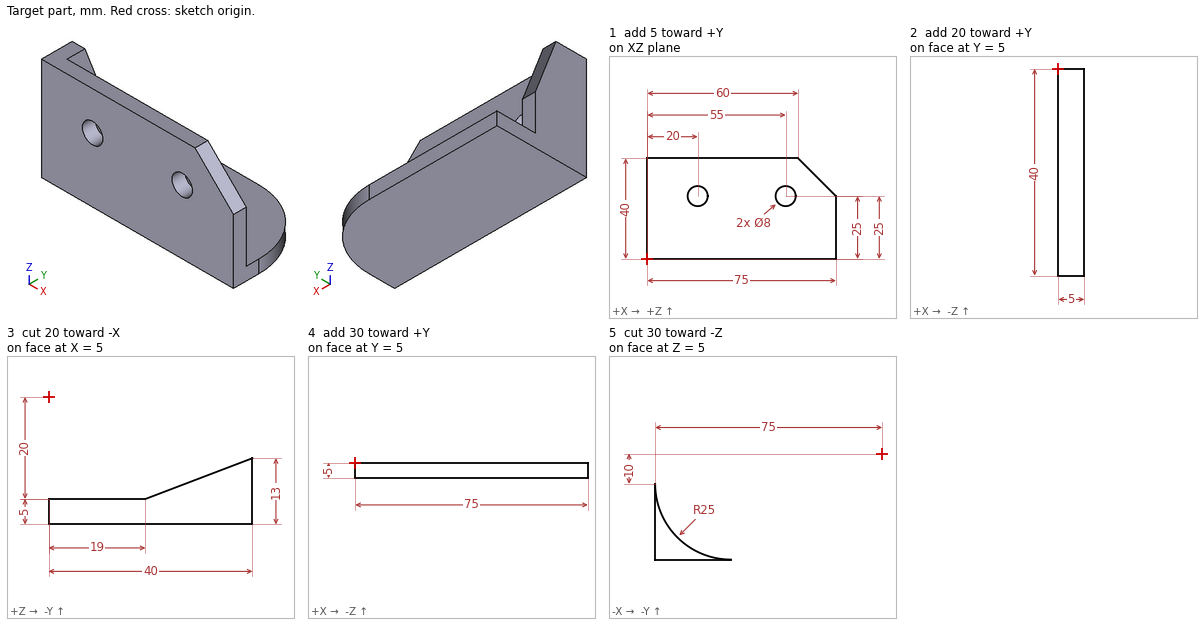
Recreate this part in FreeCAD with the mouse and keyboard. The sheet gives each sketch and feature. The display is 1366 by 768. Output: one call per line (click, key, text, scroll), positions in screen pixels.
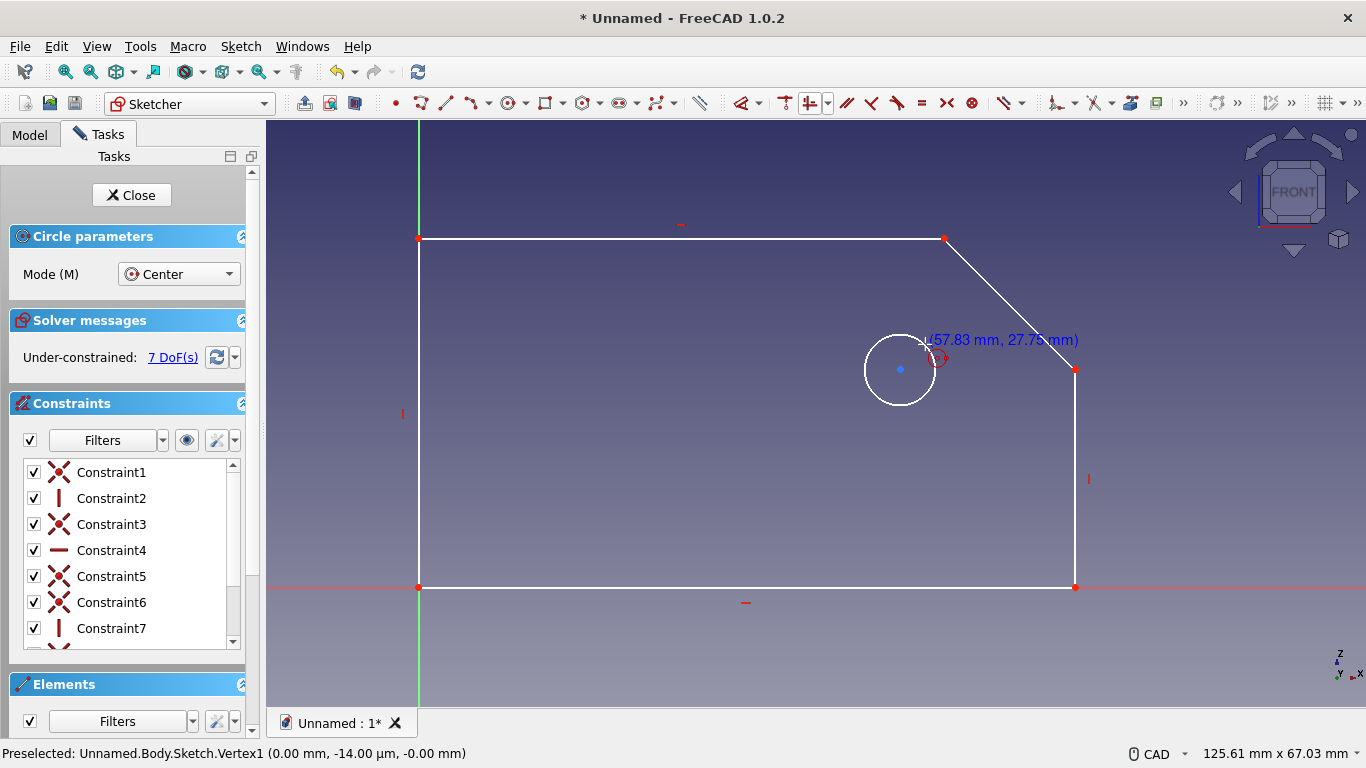
click(594, 369)
click(618, 344)
key(Escape)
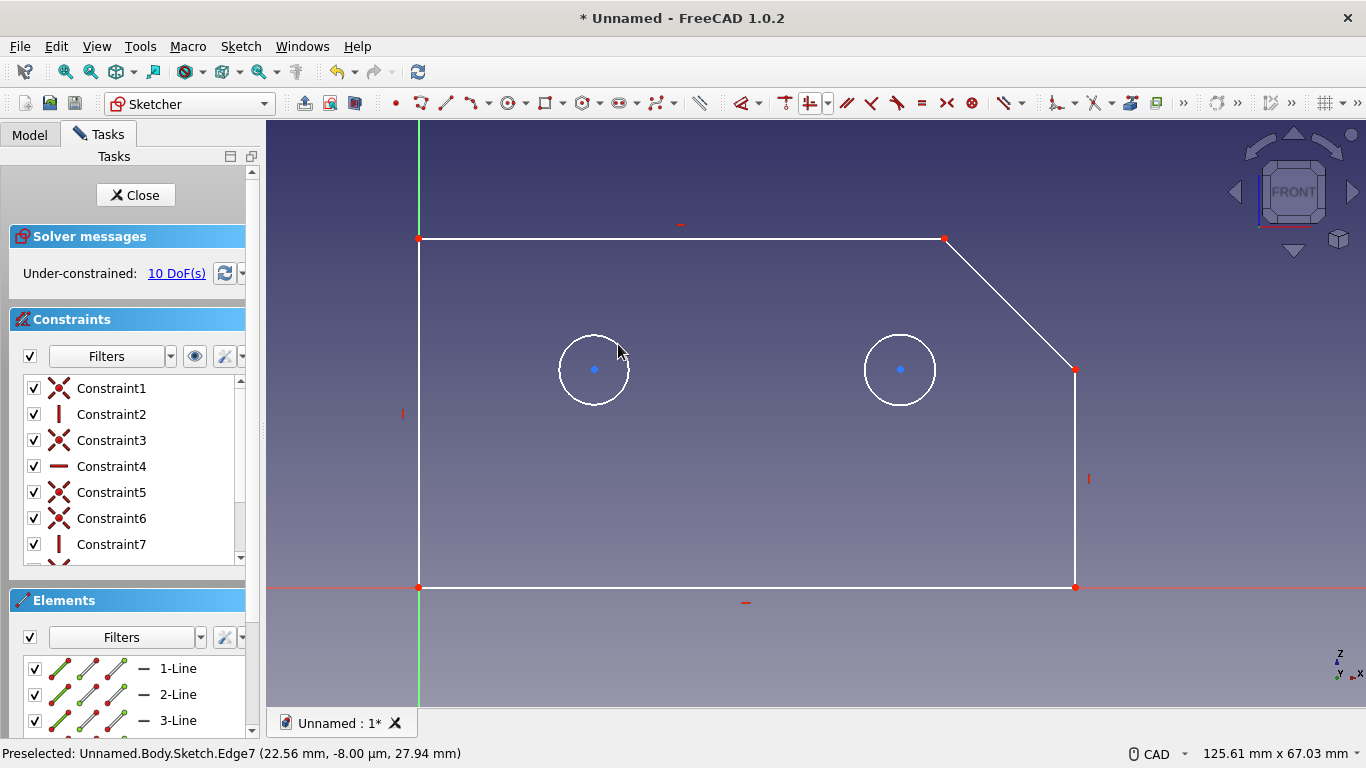
click(925, 345)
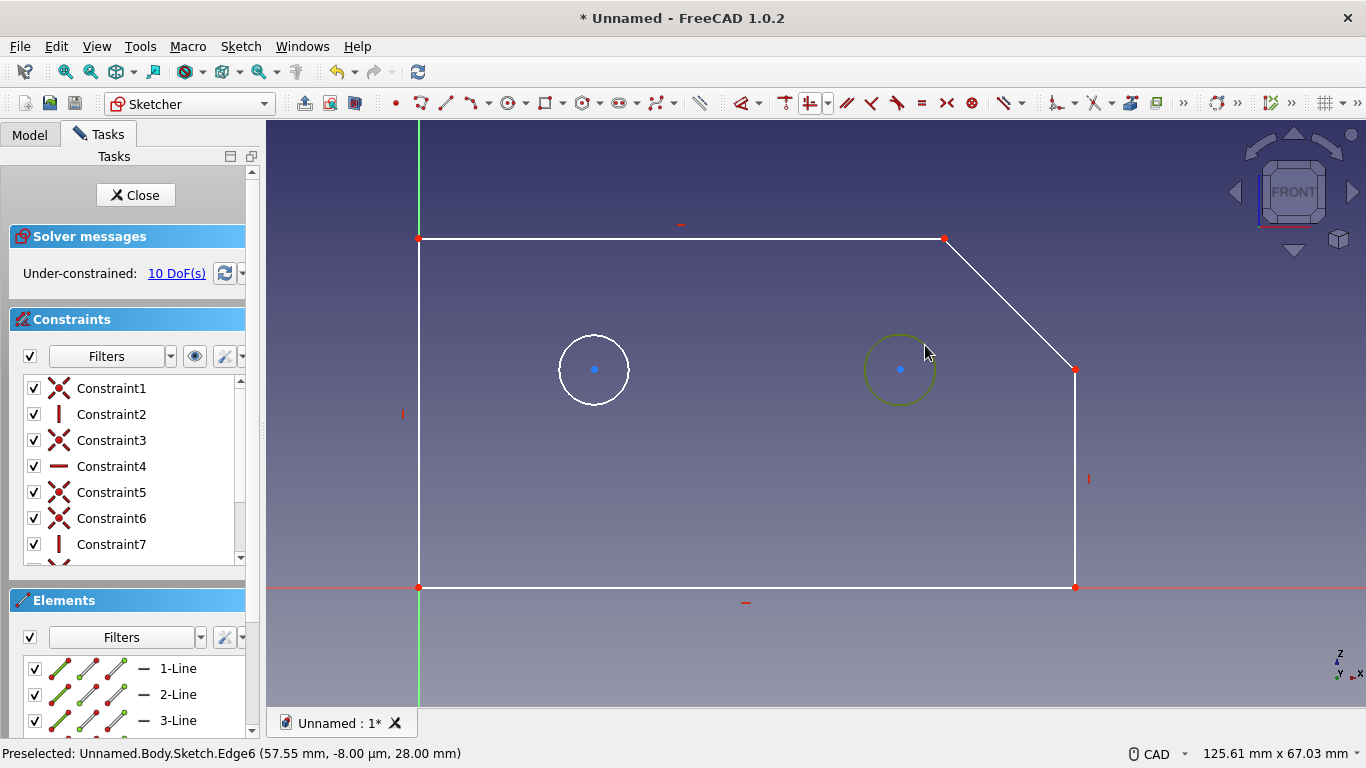
click(618, 345)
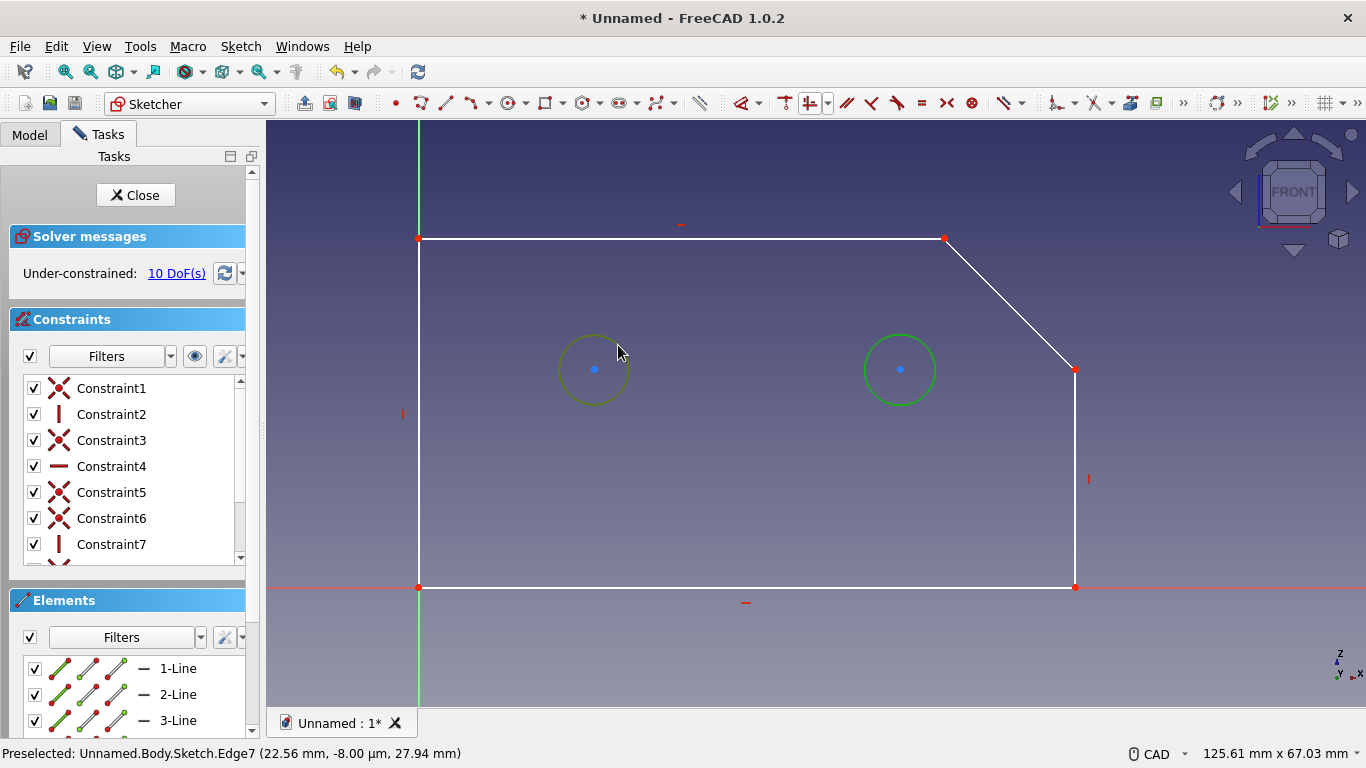
click(922, 104)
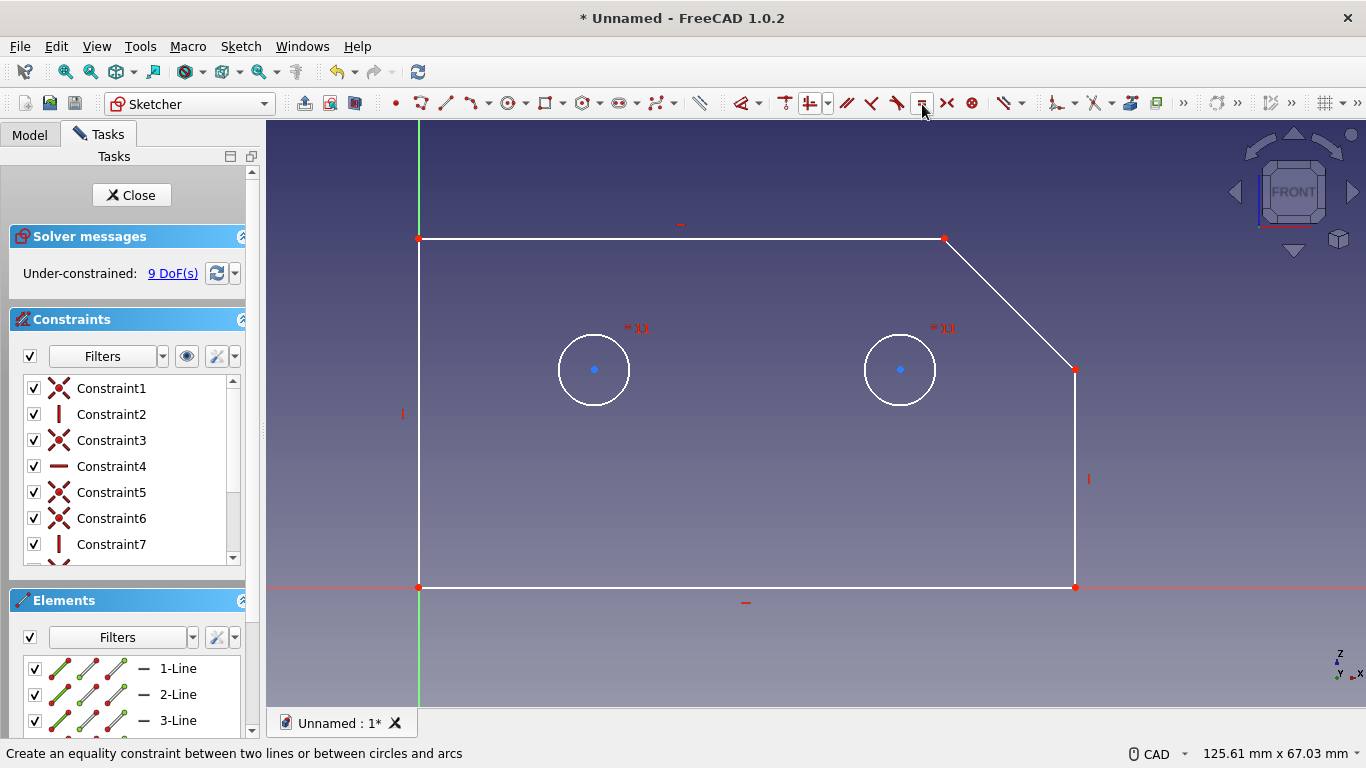
click(900, 370)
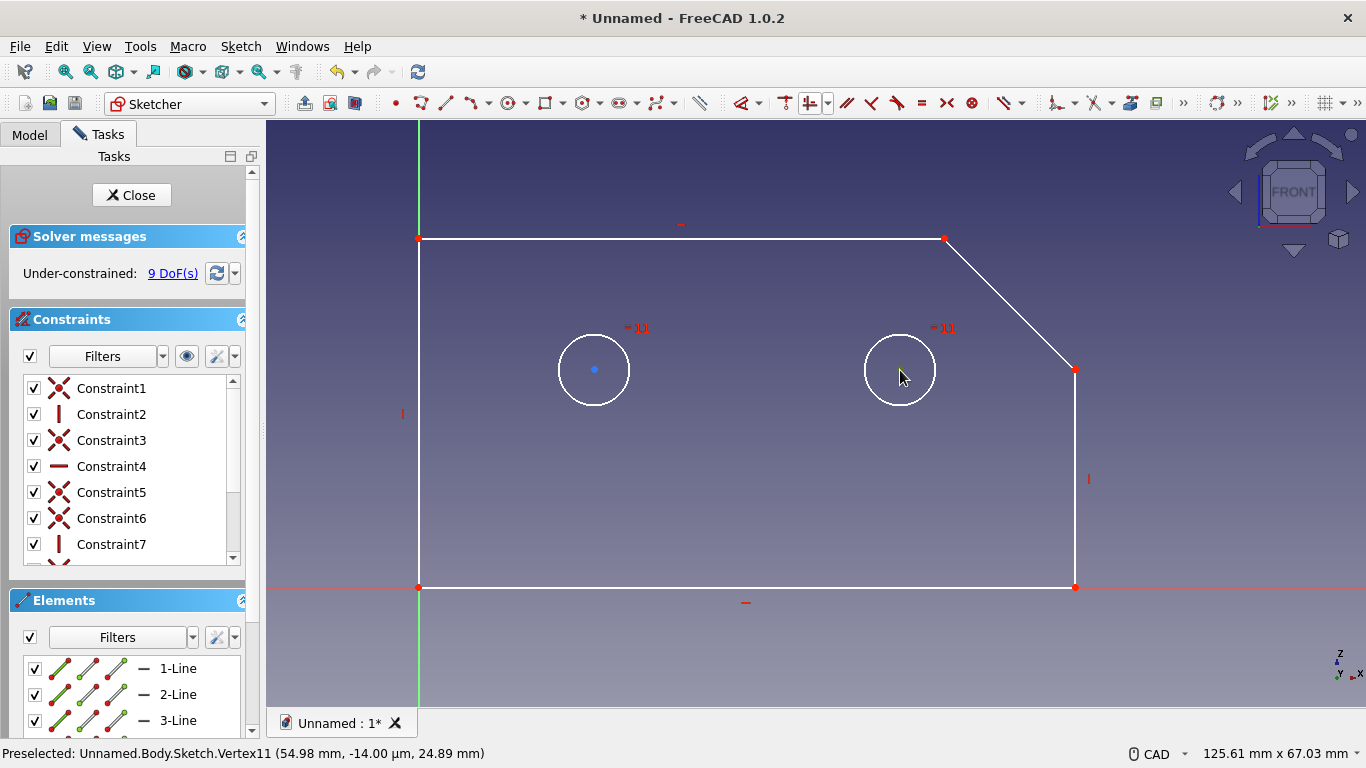
click(594, 370)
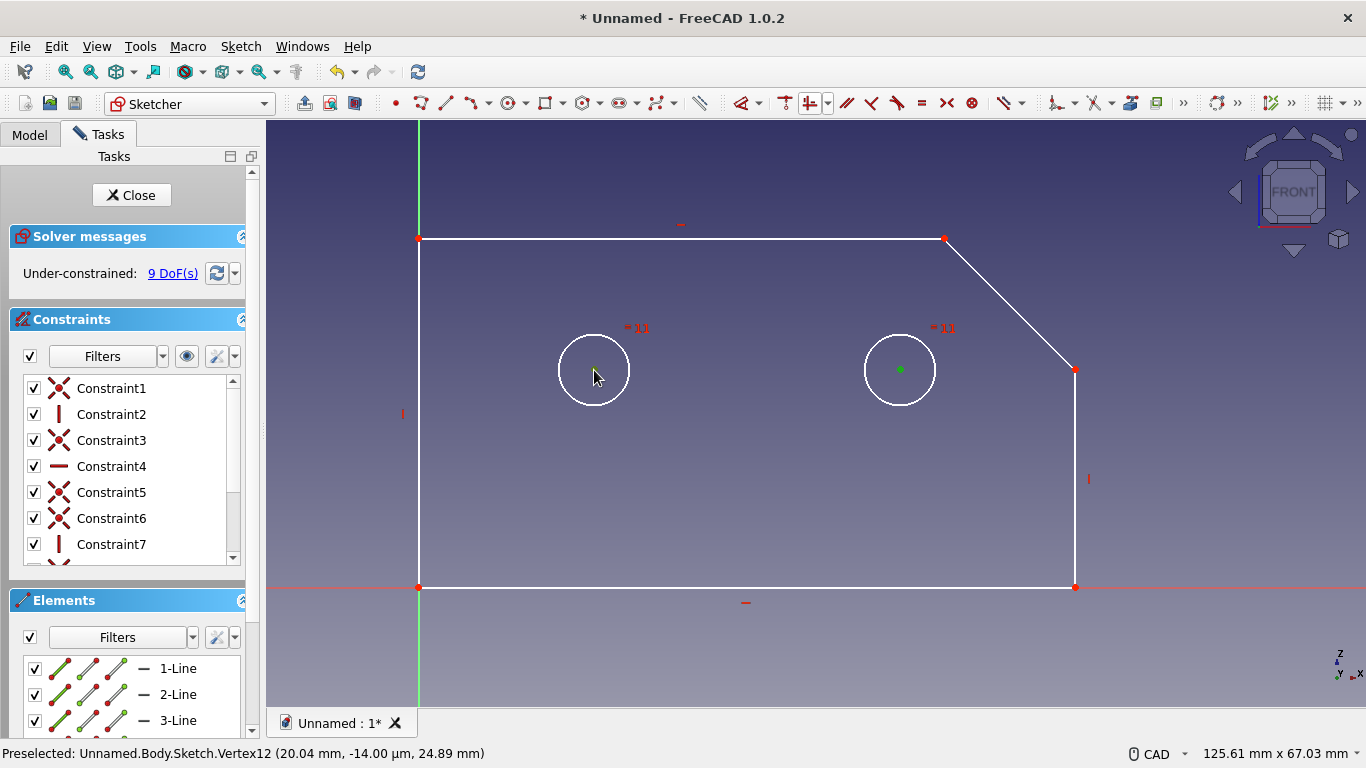
key(h)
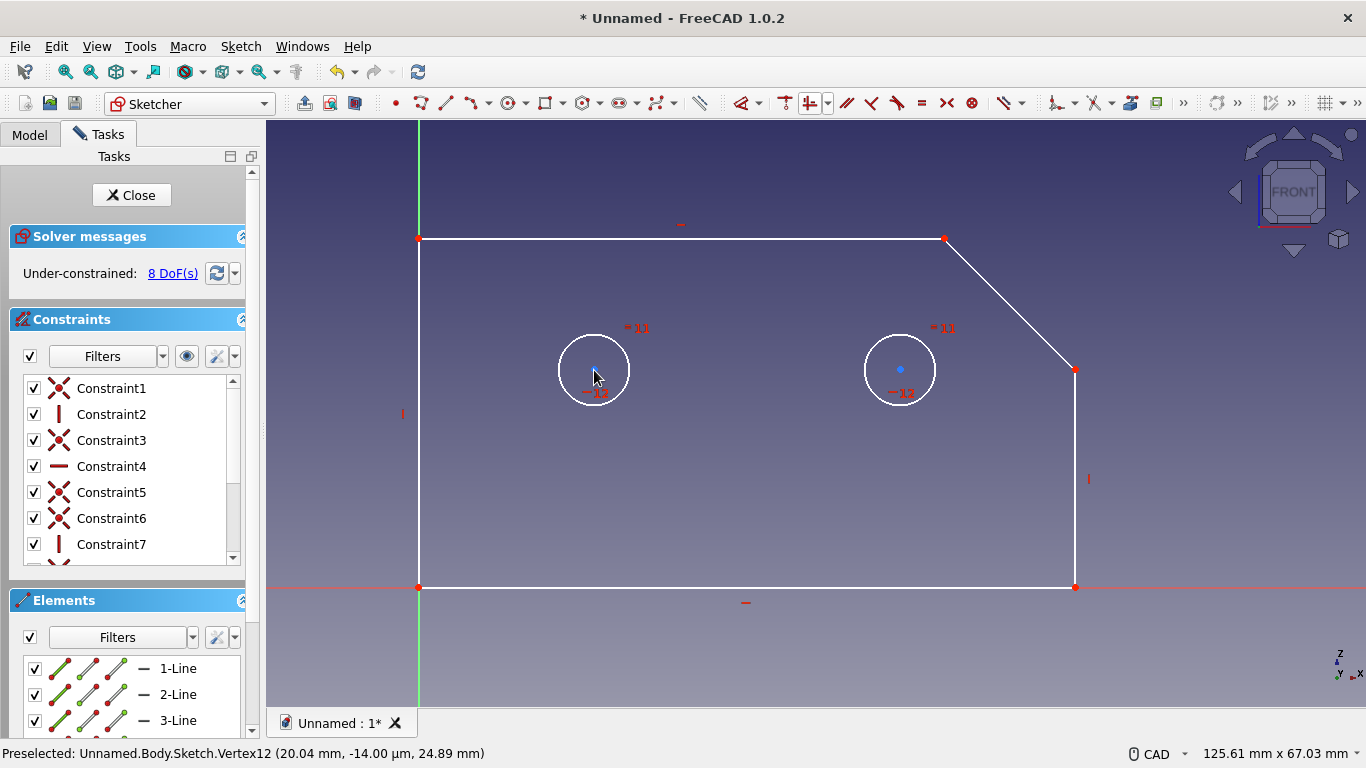
click(740, 104)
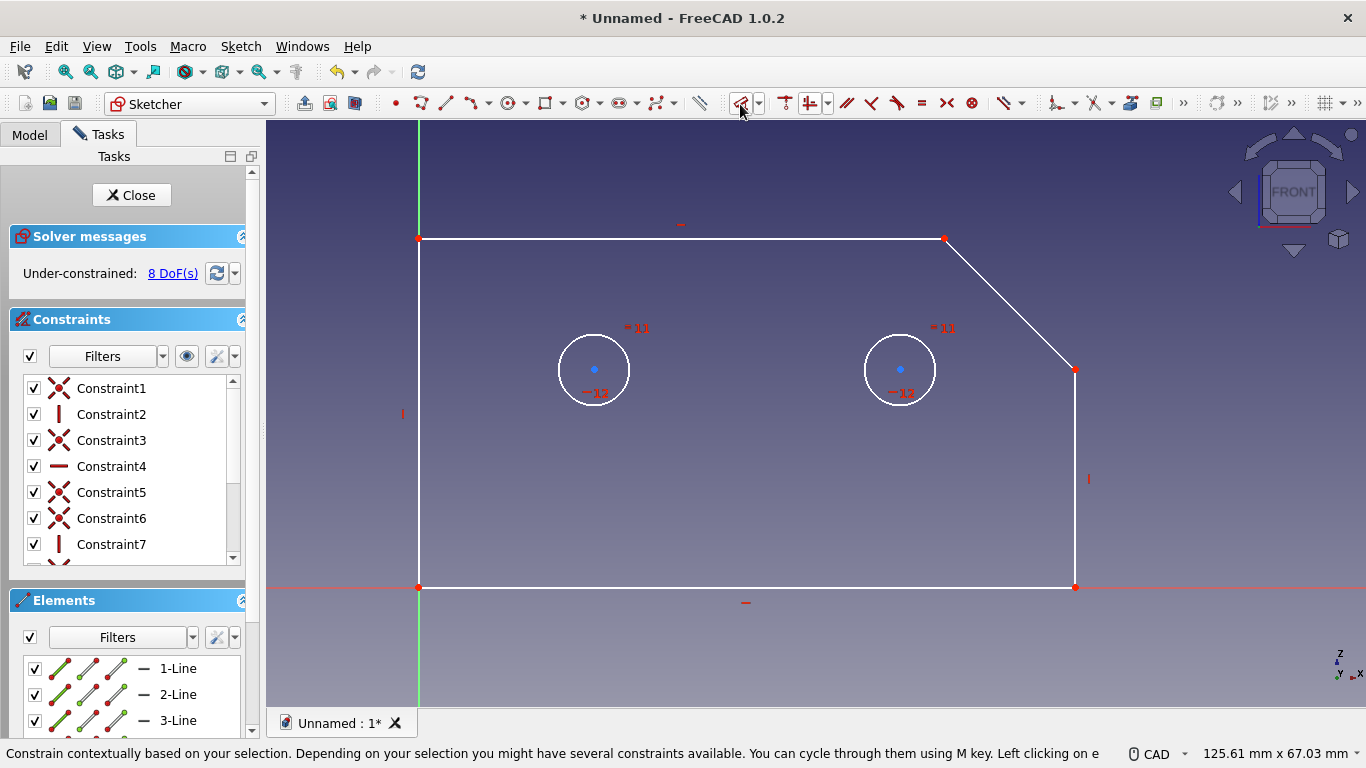
click(925, 345)
click(948, 322)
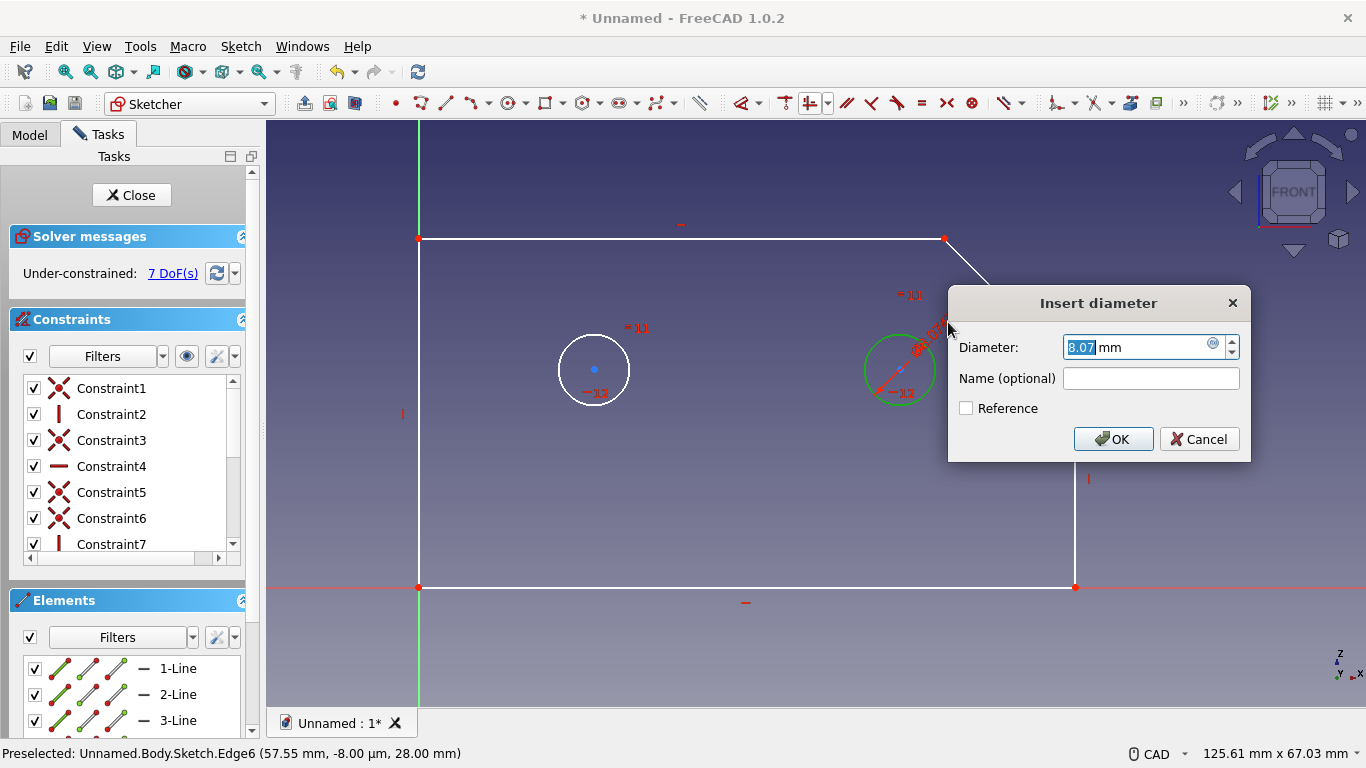
text(8)
key(Return)